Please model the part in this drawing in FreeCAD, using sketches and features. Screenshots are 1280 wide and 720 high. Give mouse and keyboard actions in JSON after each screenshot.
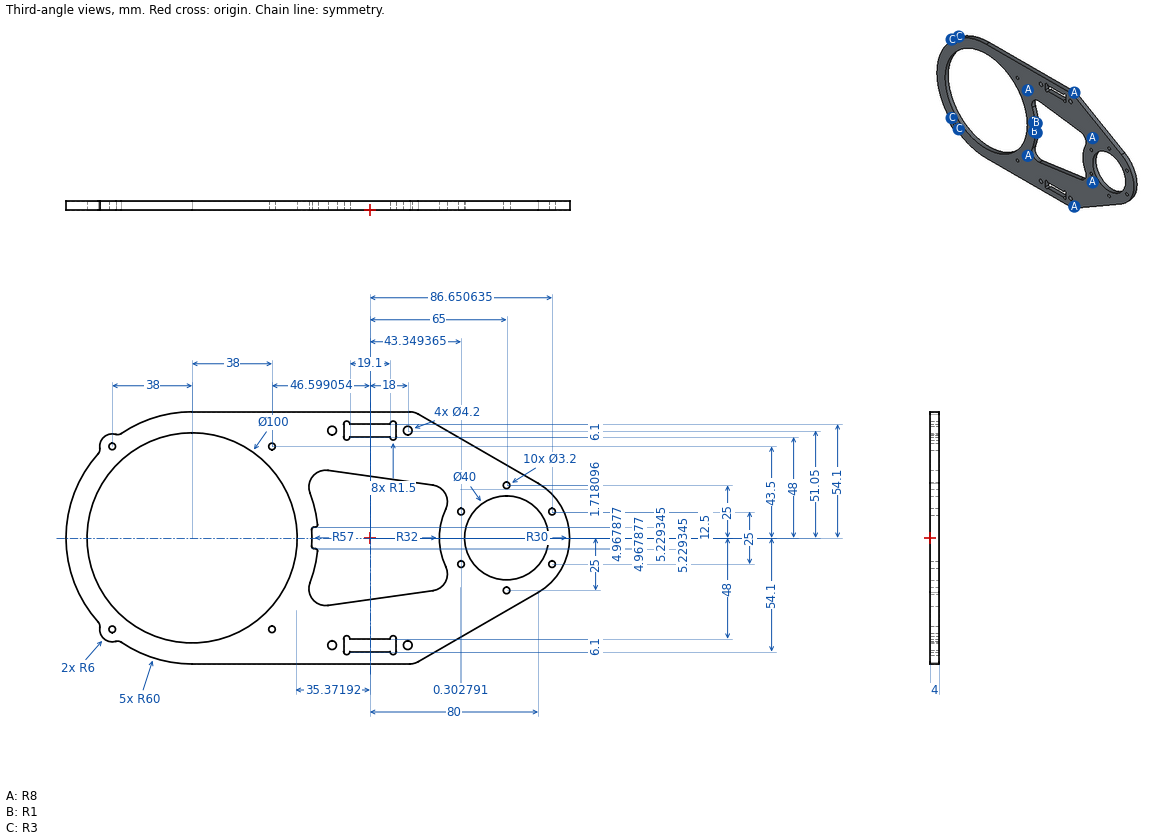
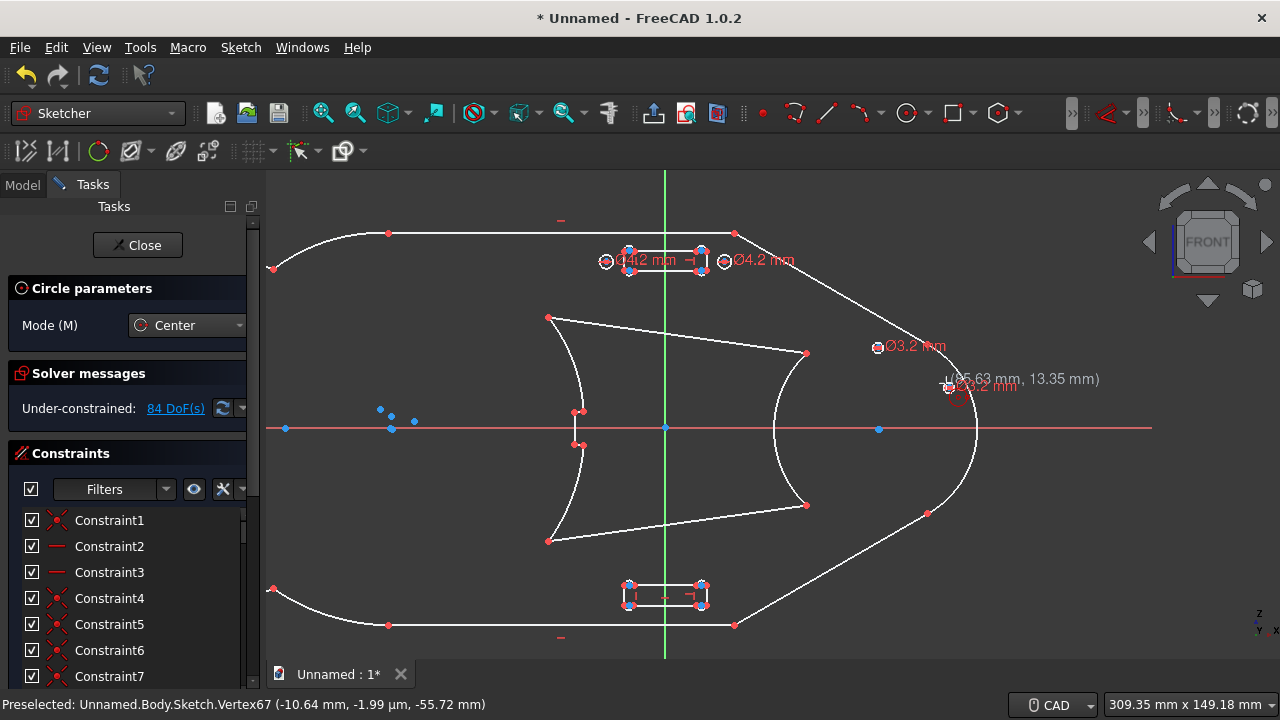
{"action": "scroll", "coordinate": [807, 387], "scroll_direction": "up", "scroll_amount": 8}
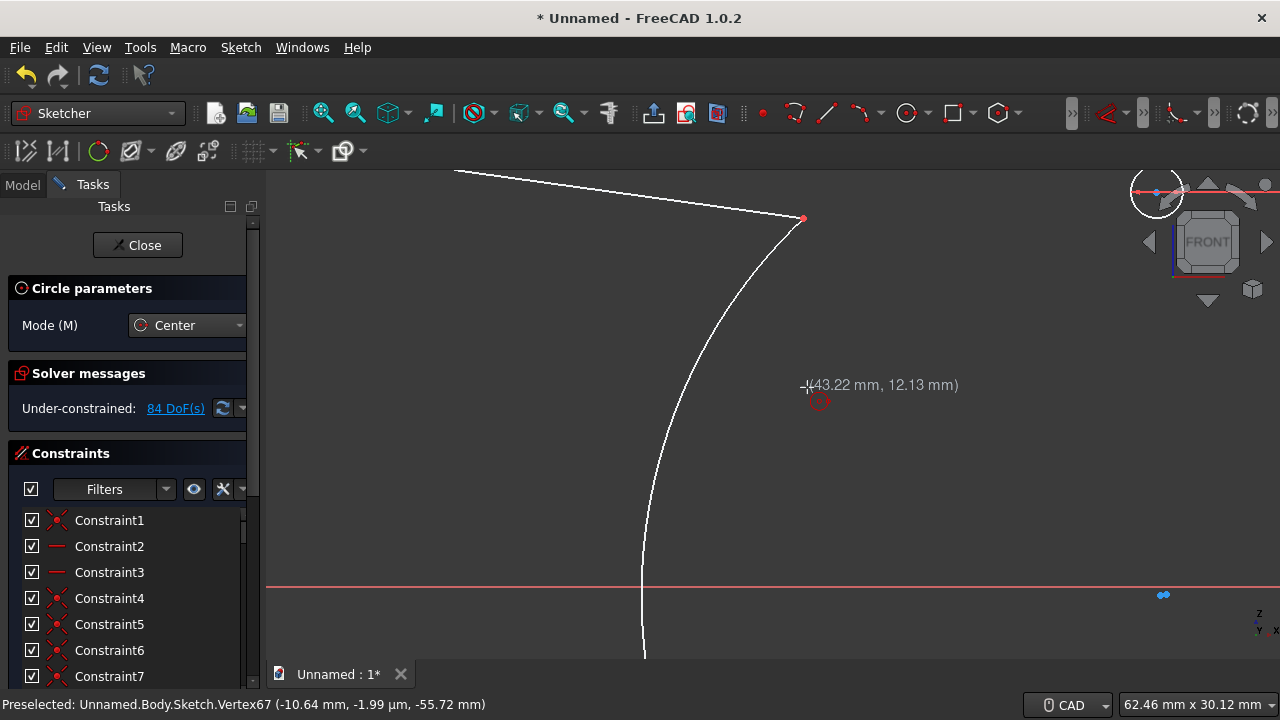
{"action": "scroll", "coordinate": [862, 387], "scroll_direction": "down", "scroll_amount": 10}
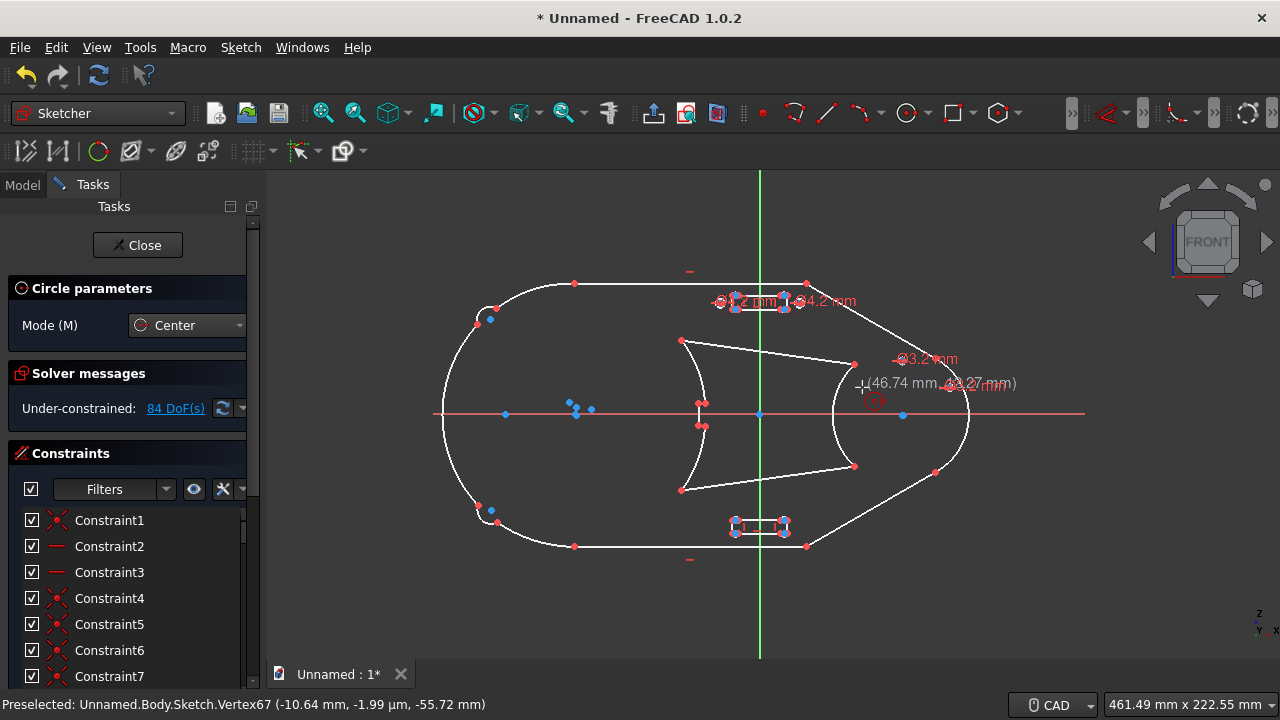
{"action": "left_click", "coordinate": [855, 387]}
{"action": "mouse_move", "coordinate": [858, 385]}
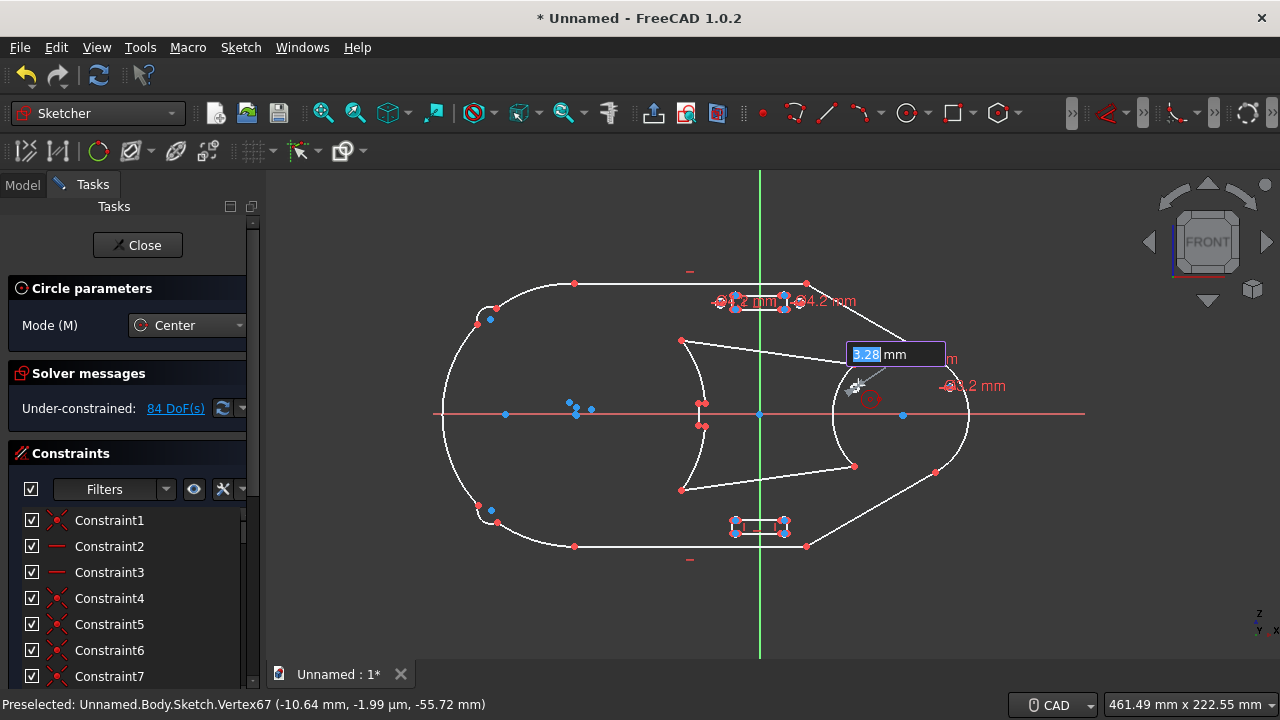
{"action": "type", "text": "3.2"}
{"action": "key", "text": "Return"}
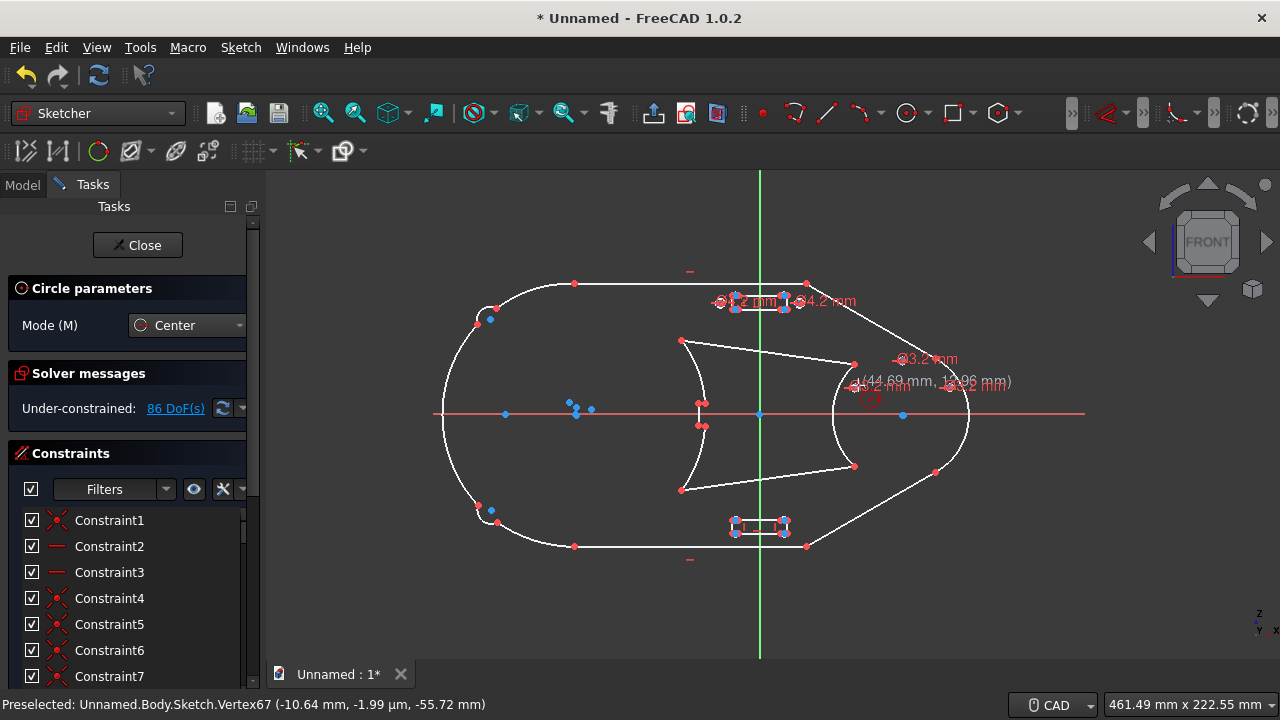
{"action": "scroll", "coordinate": [657, 319], "scroll_direction": "up", "scroll_amount": 10}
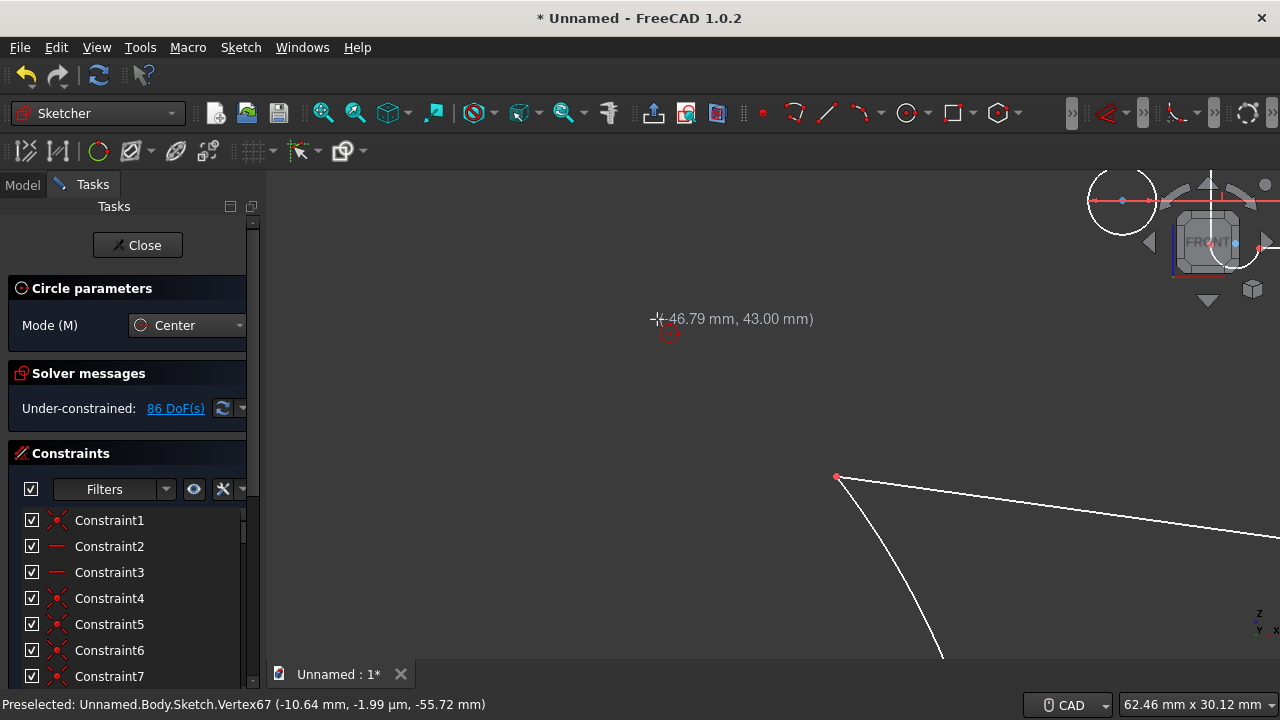
{"action": "scroll", "coordinate": [656, 319], "scroll_direction": "down", "scroll_amount": 10}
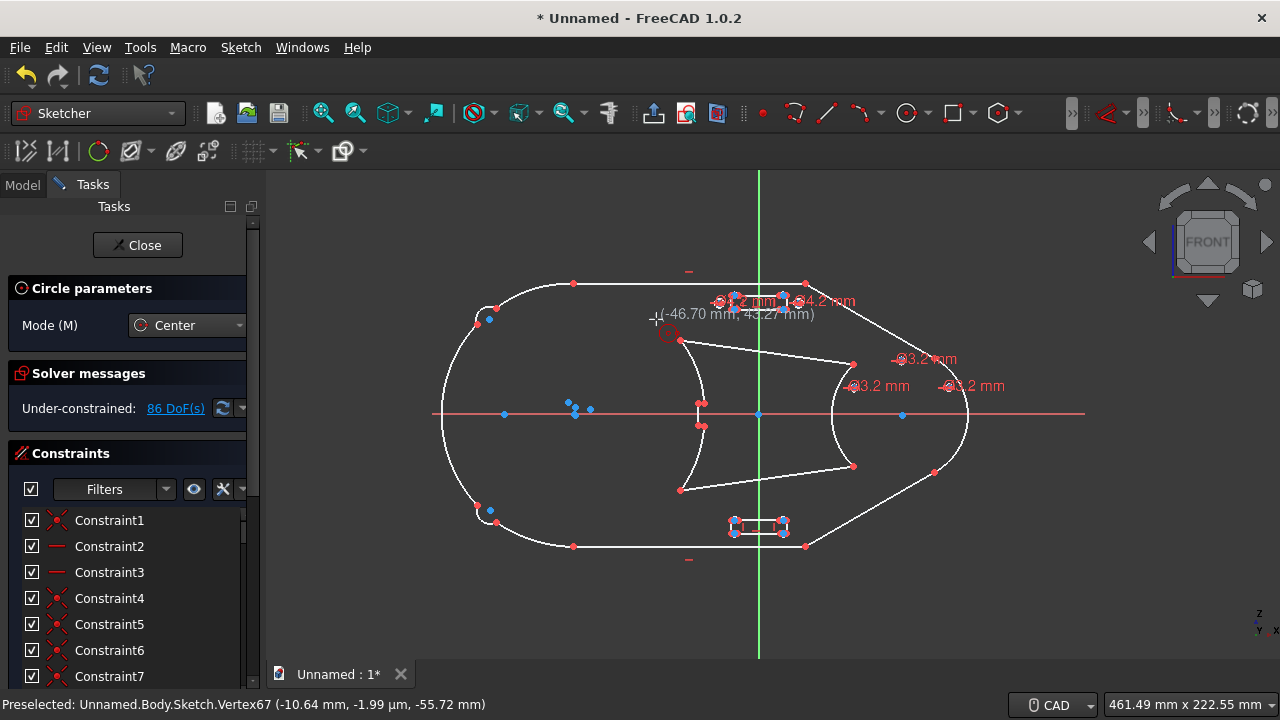
{"action": "left_click", "coordinate": [657, 319]}
{"action": "mouse_move", "coordinate": [659, 316]}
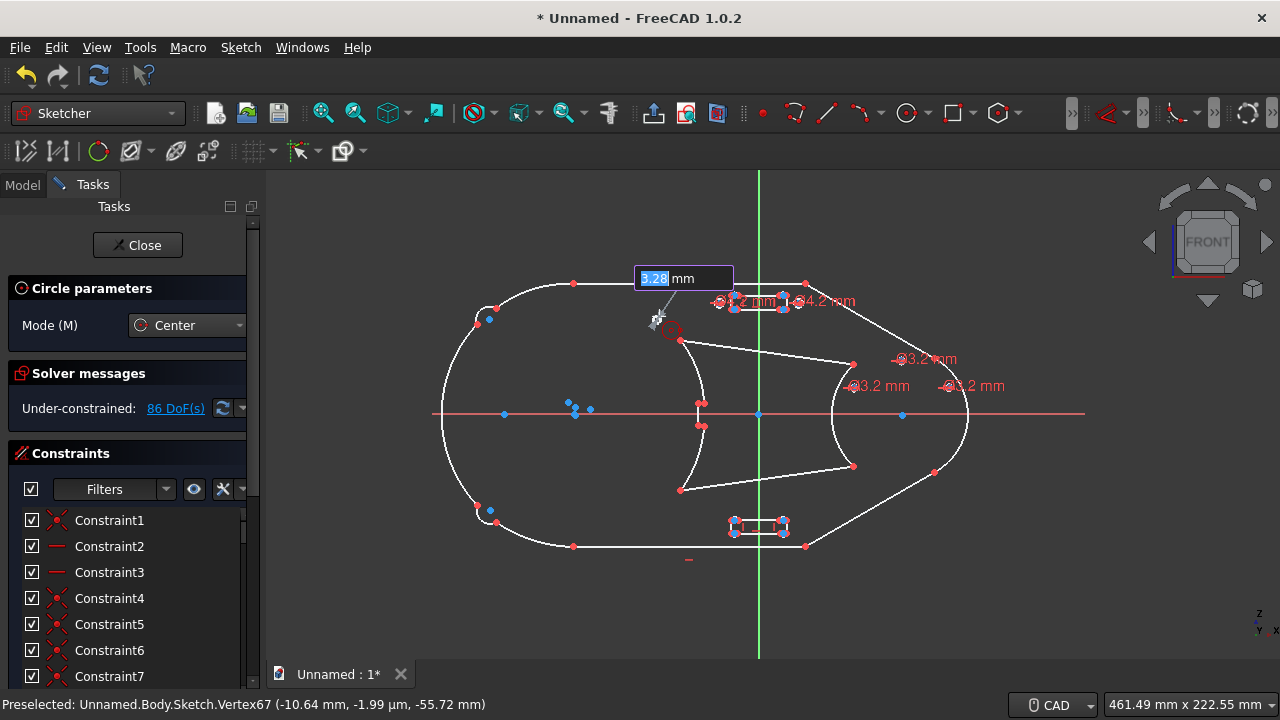
{"action": "type", "text": "3.2"}
{"action": "key", "text": "Return"}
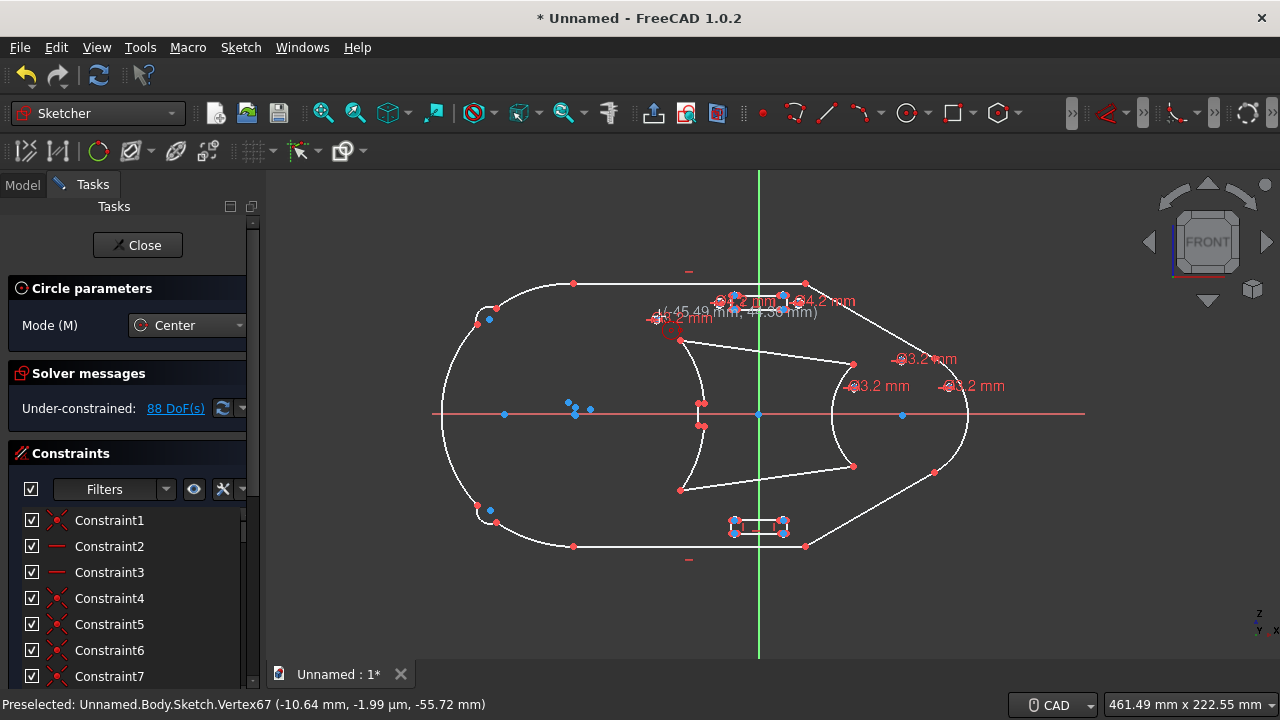
{"action": "scroll", "coordinate": [490, 319], "scroll_direction": "up", "scroll_amount": 10}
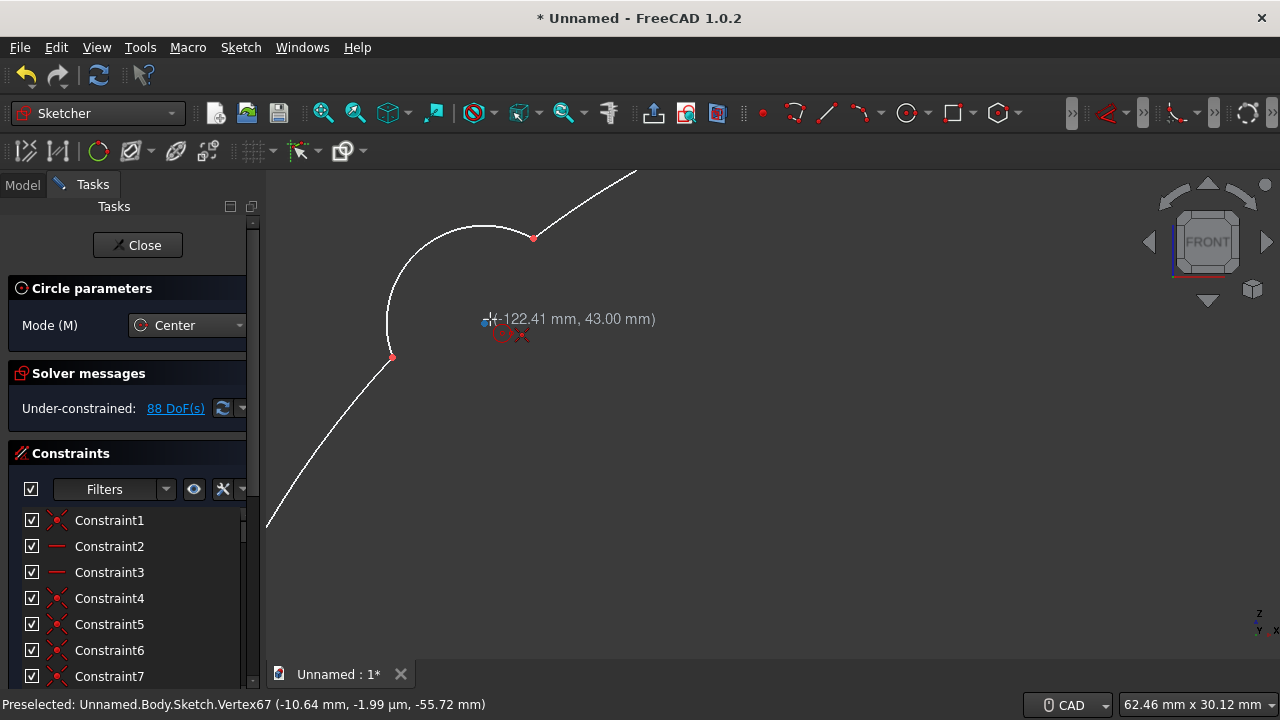
{"action": "scroll", "coordinate": [490, 319], "scroll_direction": "down", "scroll_amount": 10}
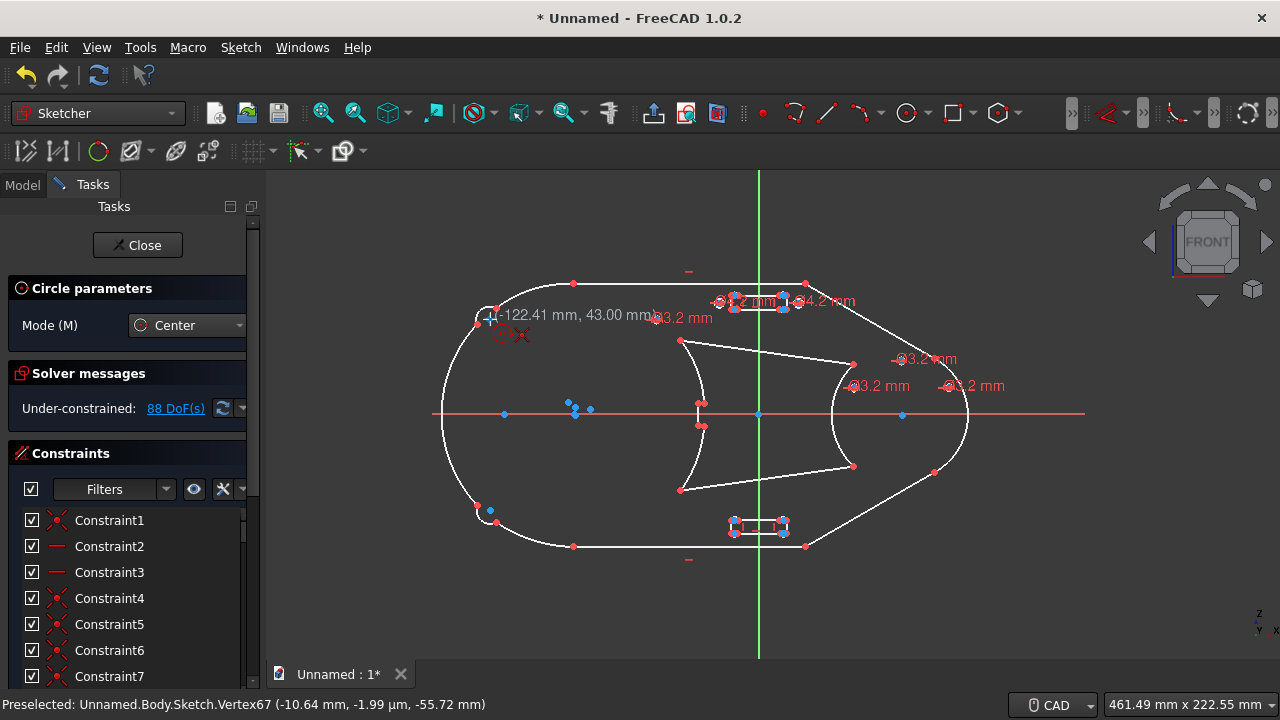
{"action": "left_click", "coordinate": [490, 319]}